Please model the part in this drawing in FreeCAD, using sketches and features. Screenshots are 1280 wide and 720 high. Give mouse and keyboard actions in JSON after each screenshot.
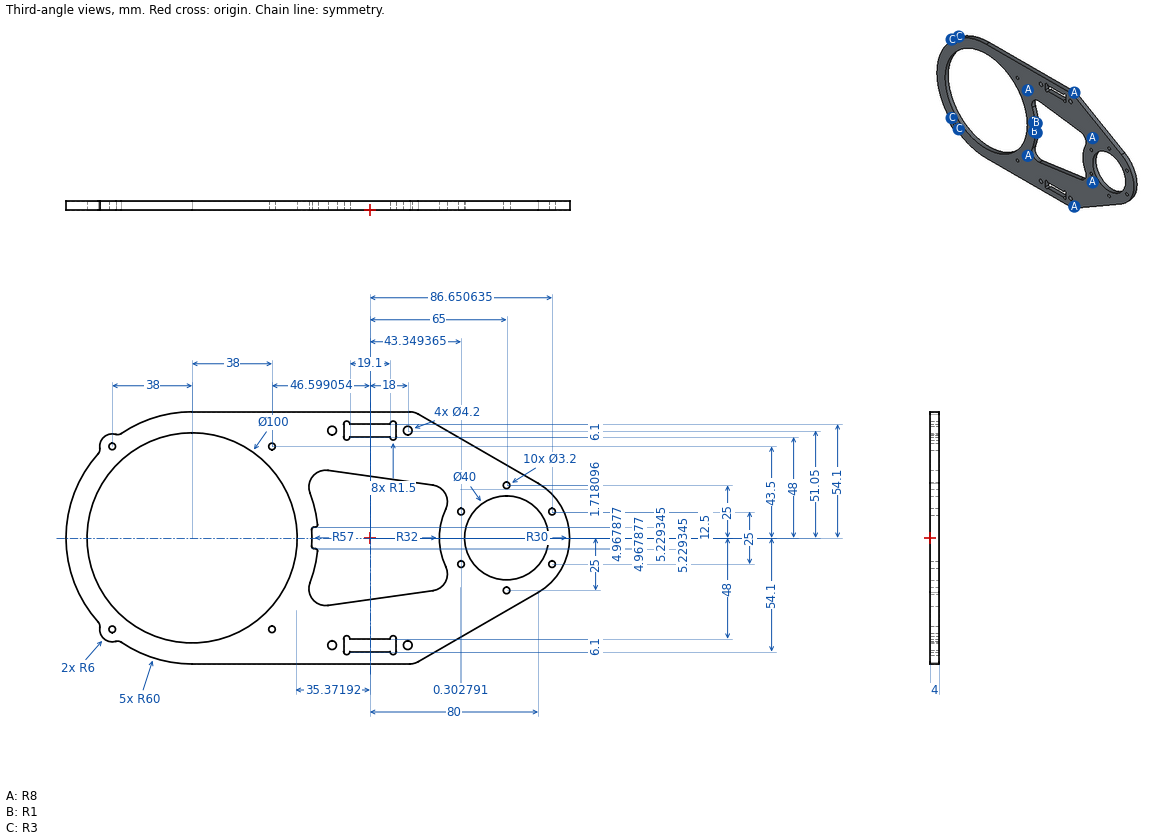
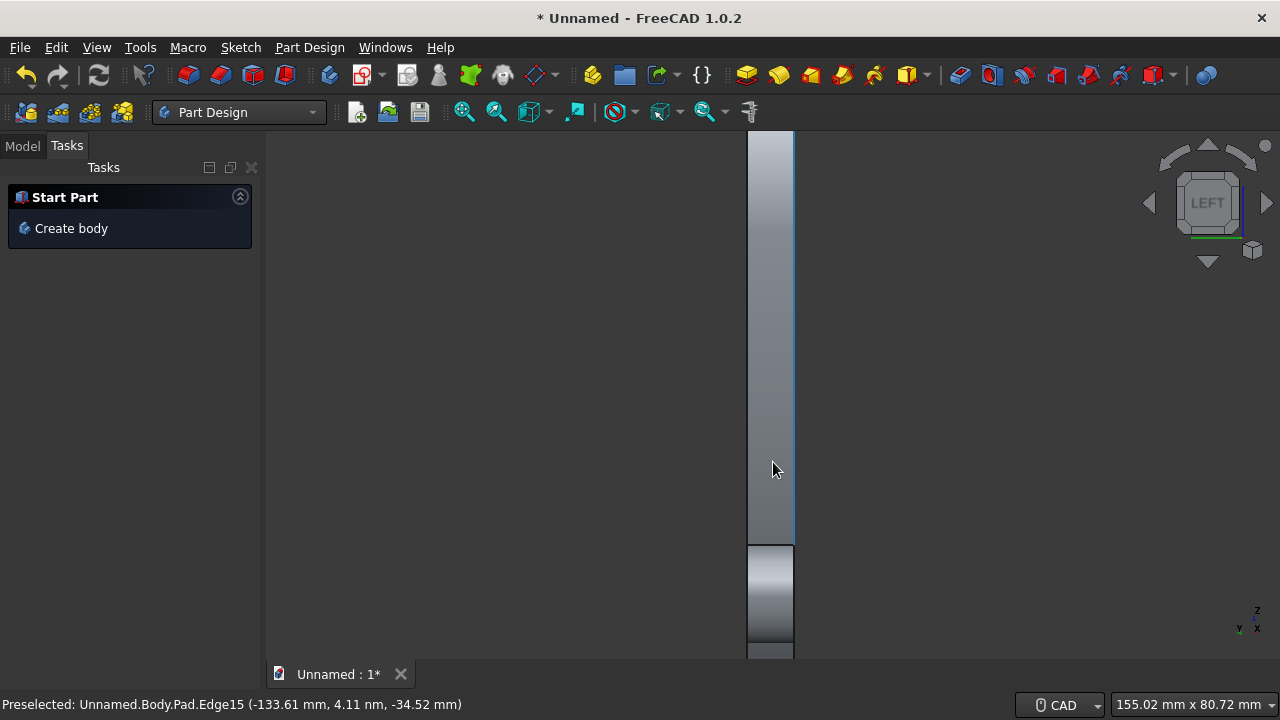
{"action": "left_click", "coordinate": [466, 112]}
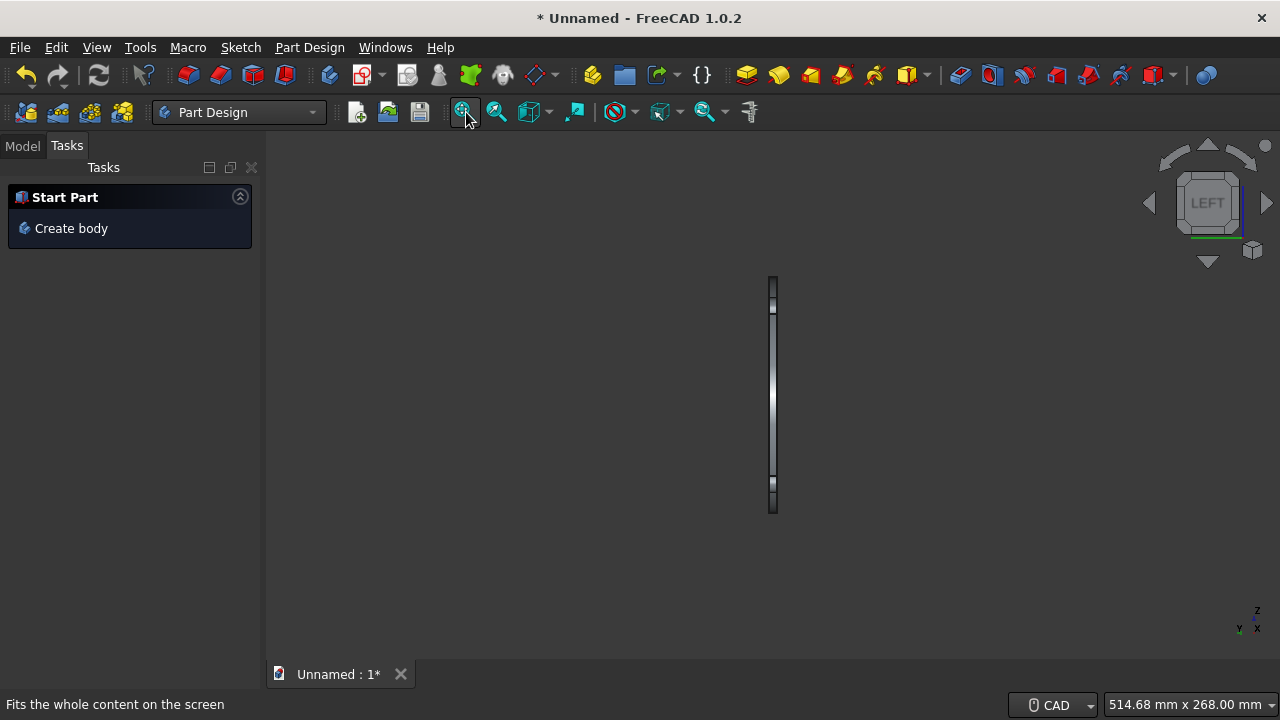
{"action": "key", "text": "v 3"}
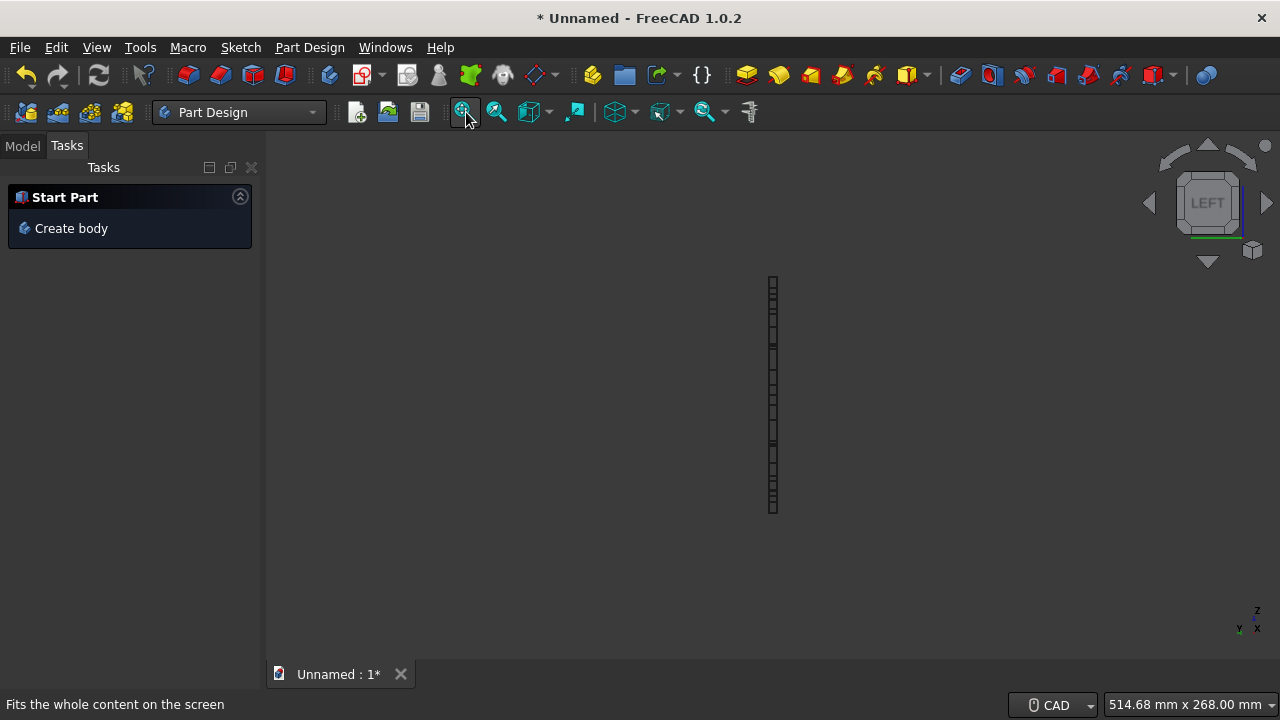
{"action": "key", "text": "0"}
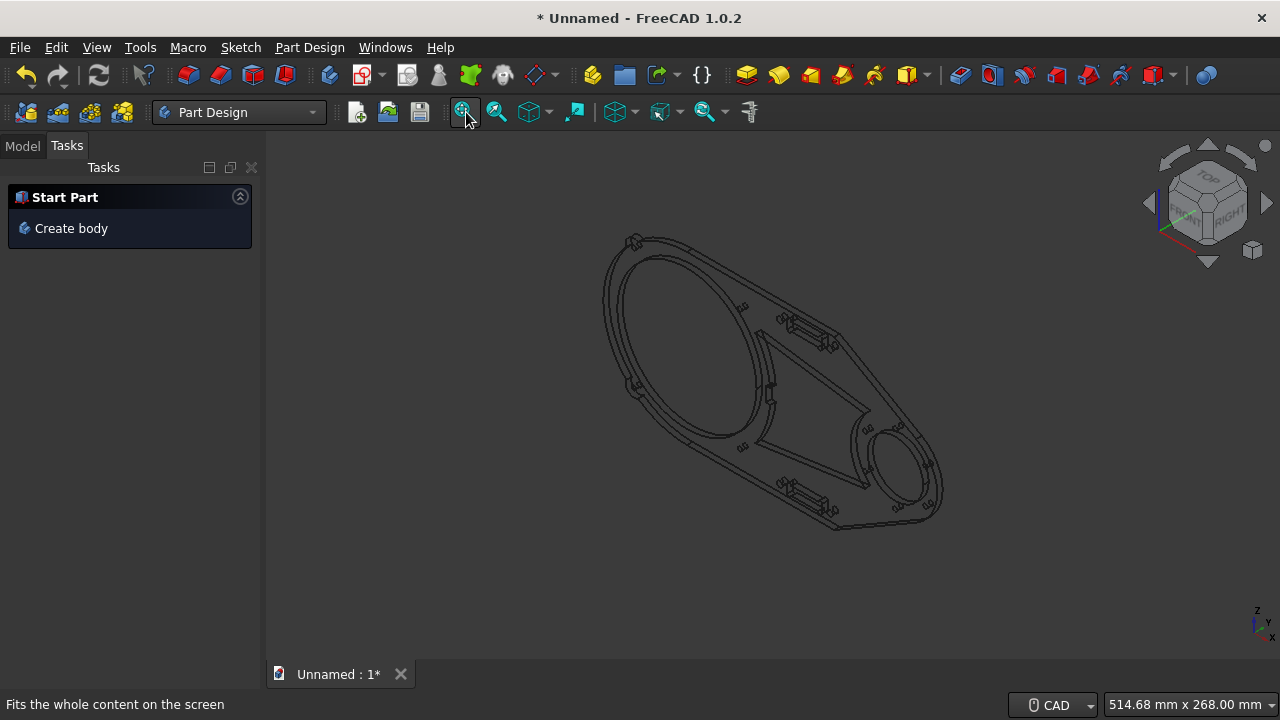
{"action": "scroll", "coordinate": [758, 441], "scroll_direction": "up", "scroll_amount": 9}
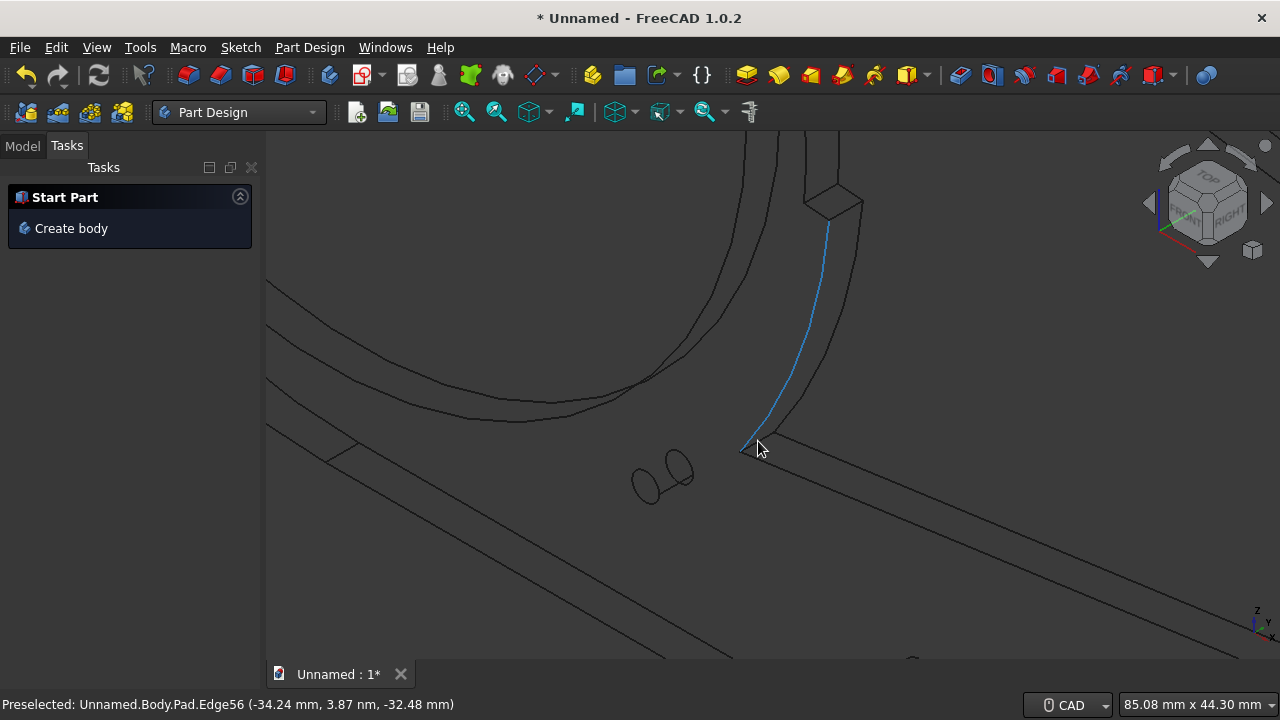
{"action": "left_click", "coordinate": [757, 441]}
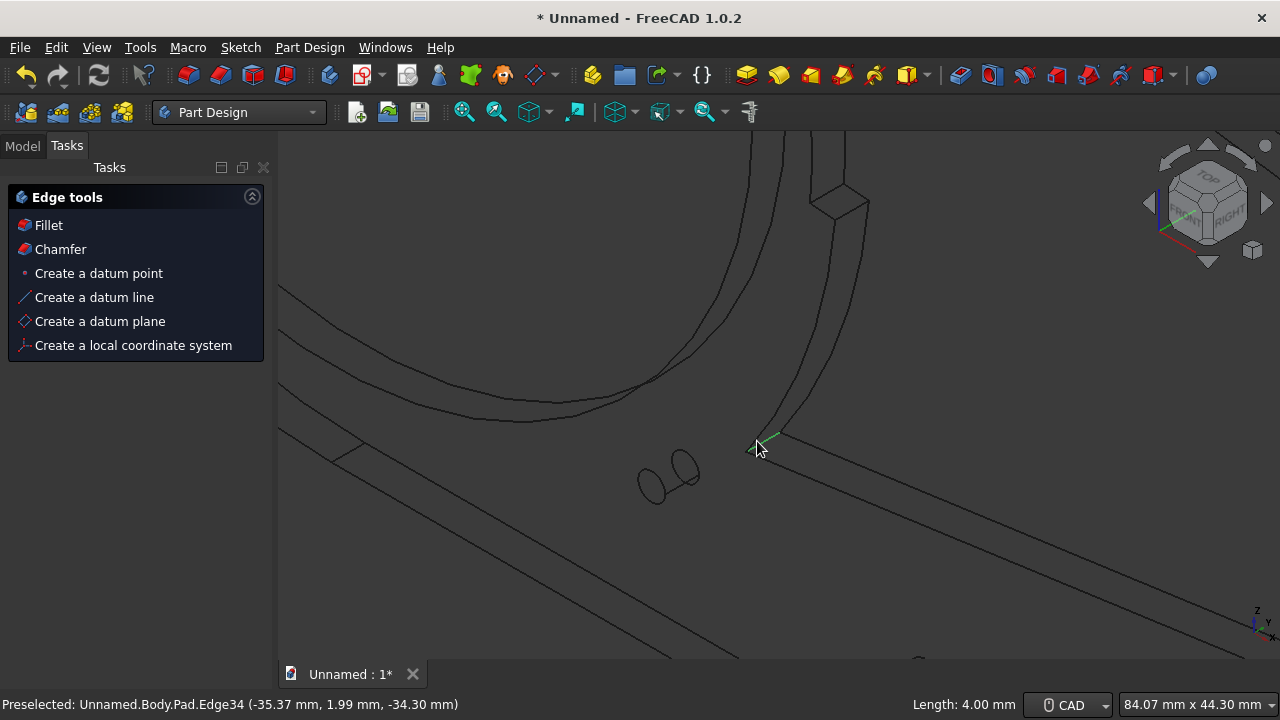
{"action": "key", "text": "v f"}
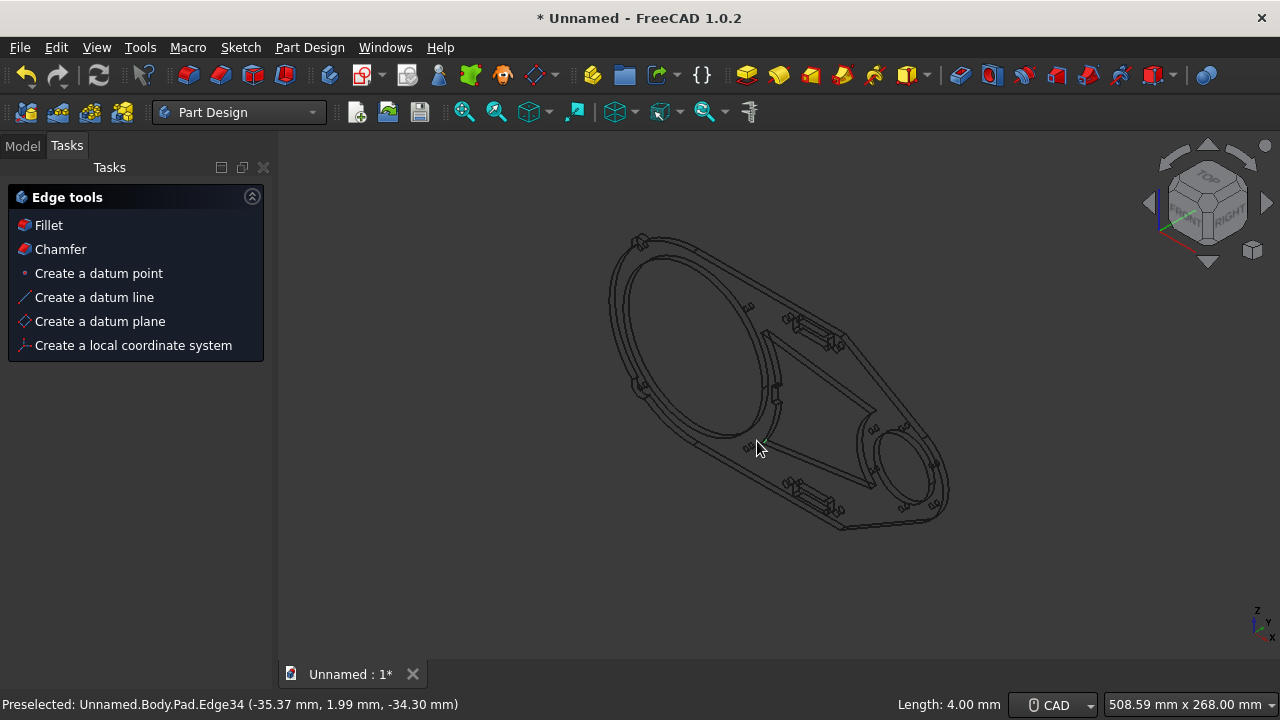
{"action": "key", "text": "2"}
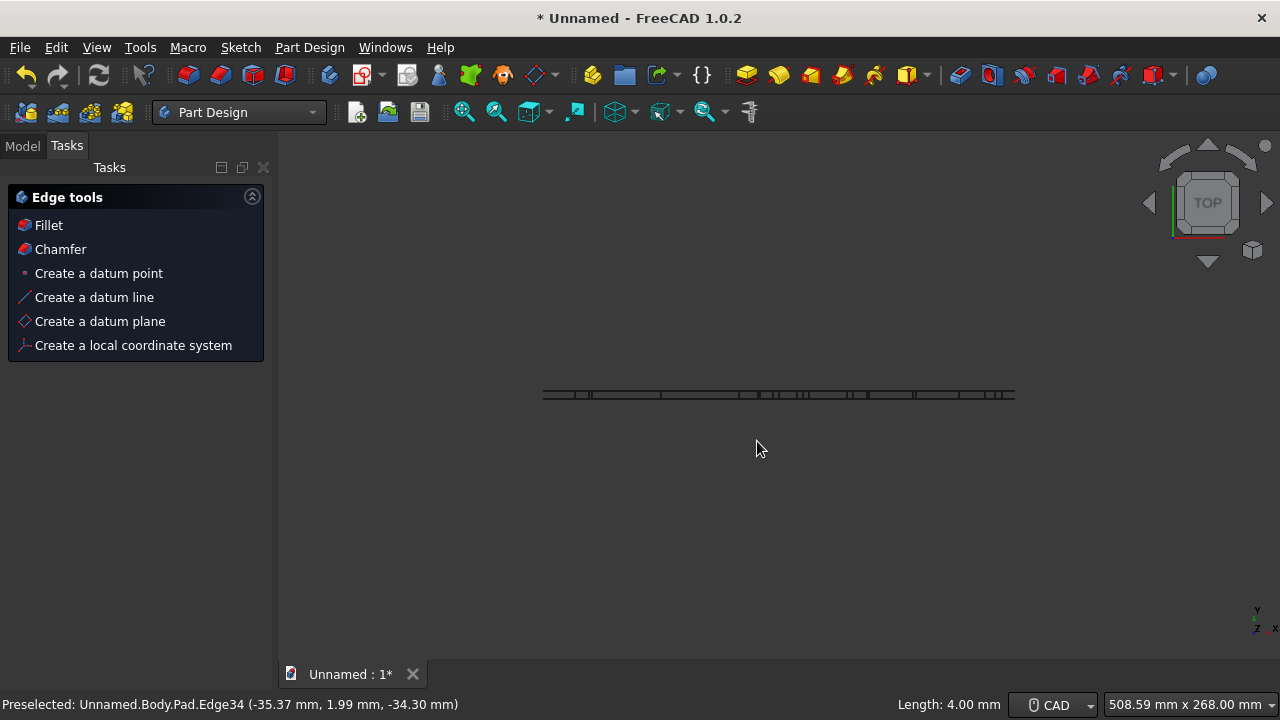
{"action": "left_click", "coordinate": [869, 397], "text": "ctrl"}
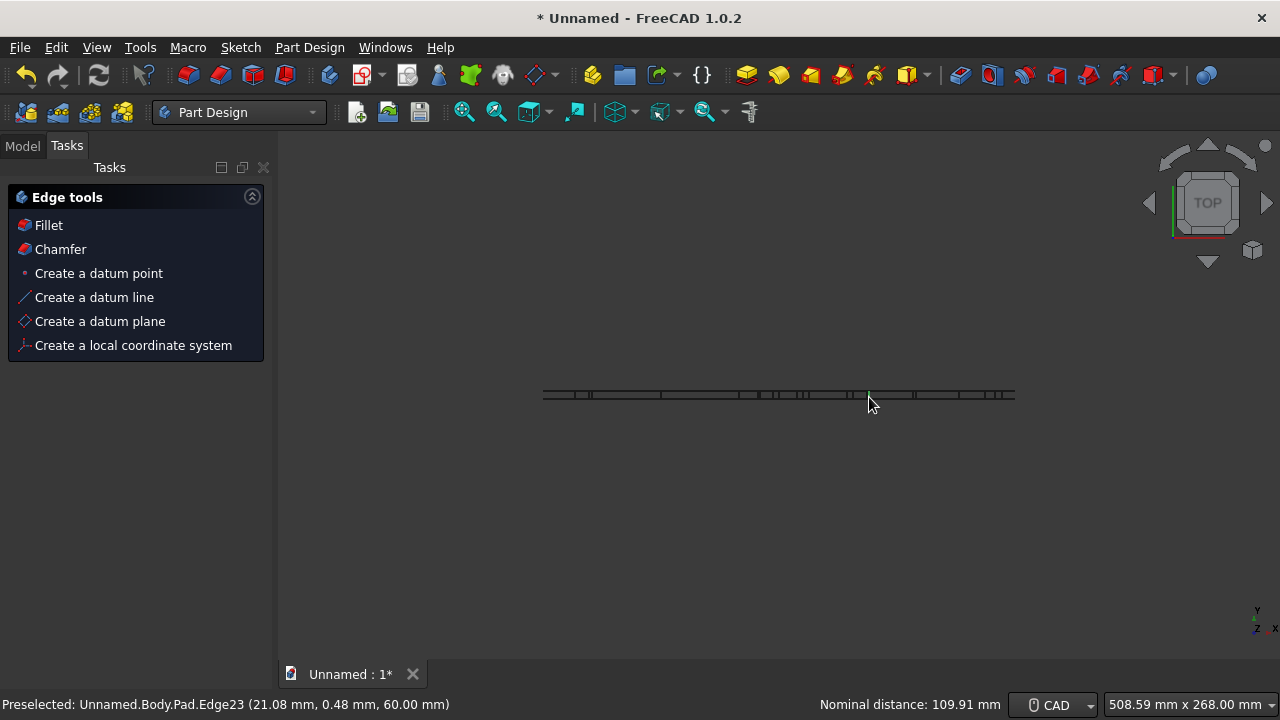
{"action": "scroll", "coordinate": [758, 394], "scroll_direction": "up", "scroll_amount": 9}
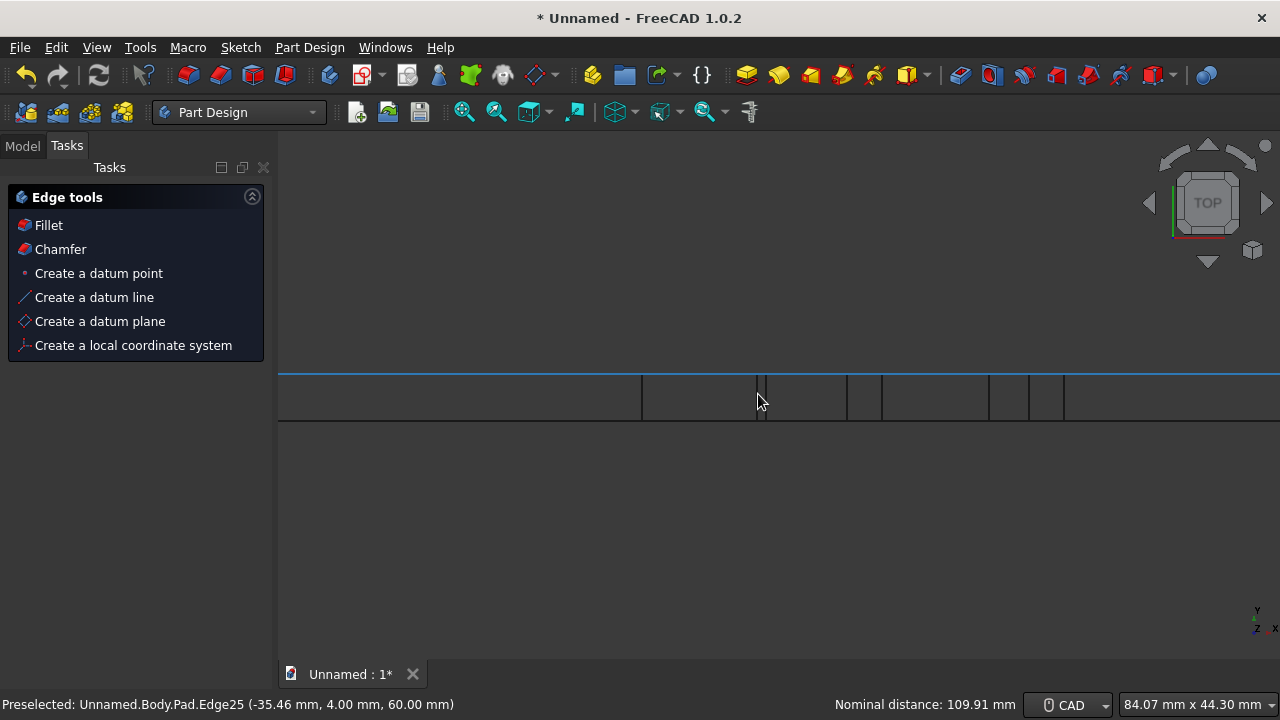
{"action": "left_click", "coordinate": [757, 397], "text": "ctrl"}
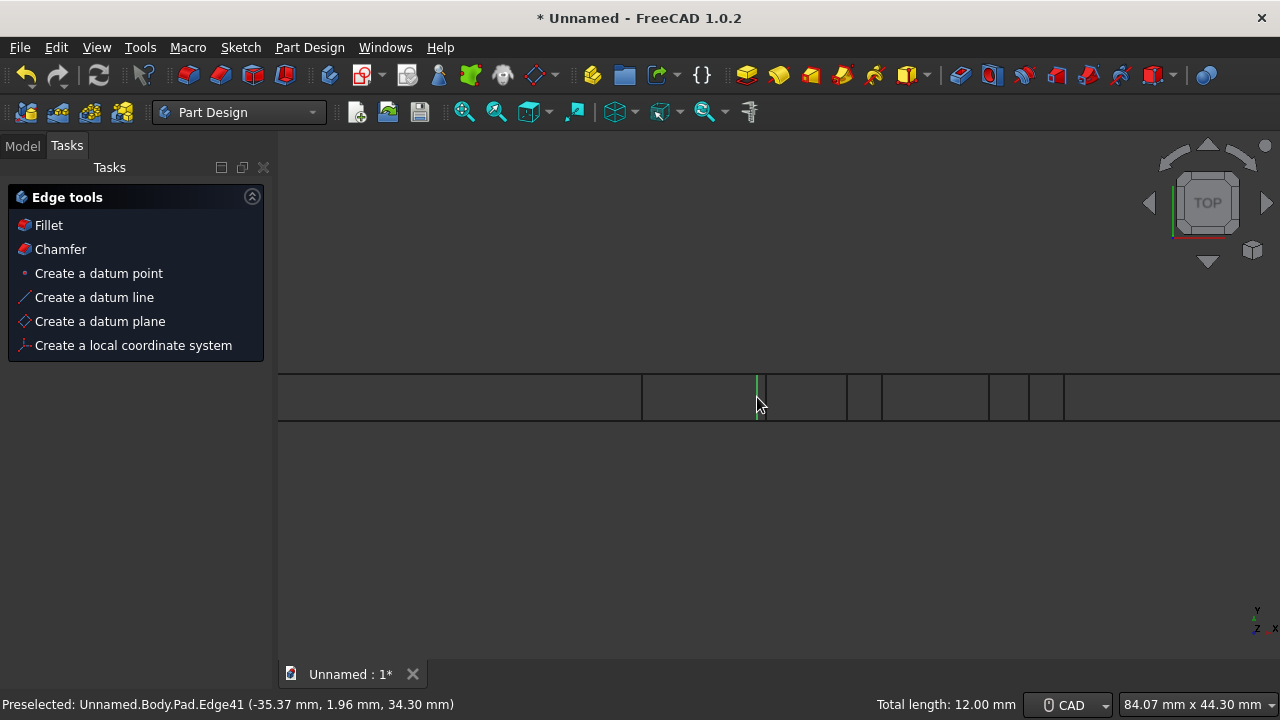
{"action": "left_click", "coordinate": [466, 112]}